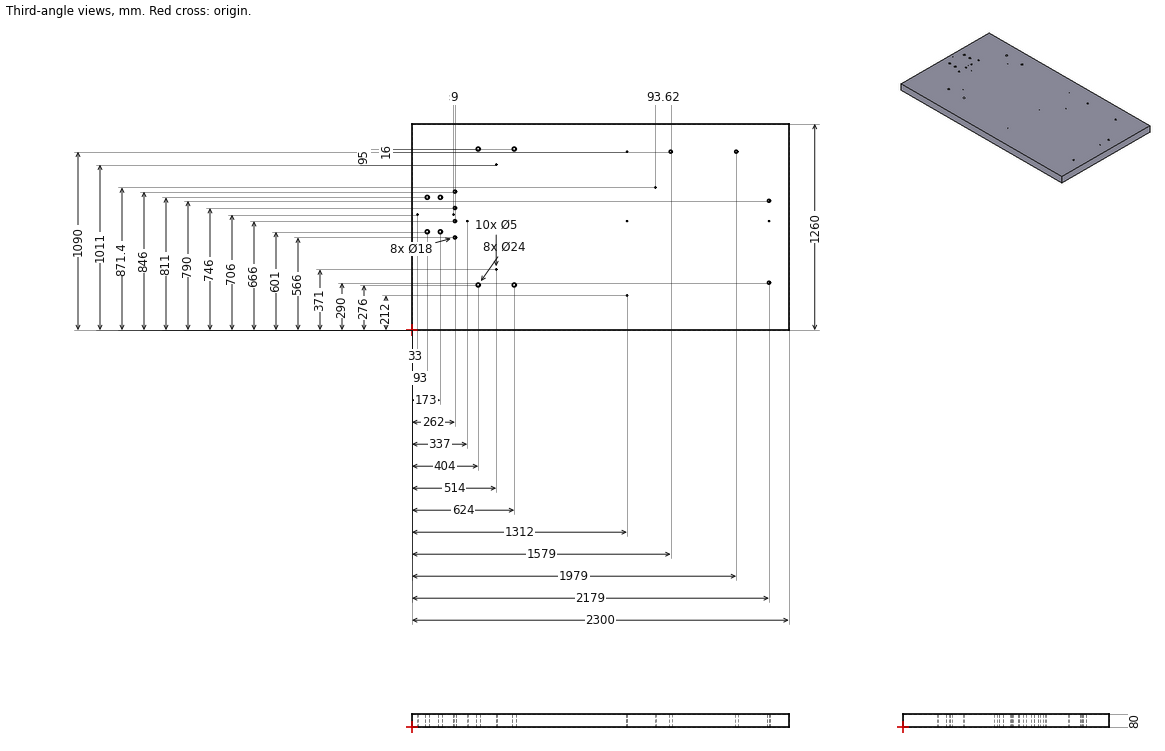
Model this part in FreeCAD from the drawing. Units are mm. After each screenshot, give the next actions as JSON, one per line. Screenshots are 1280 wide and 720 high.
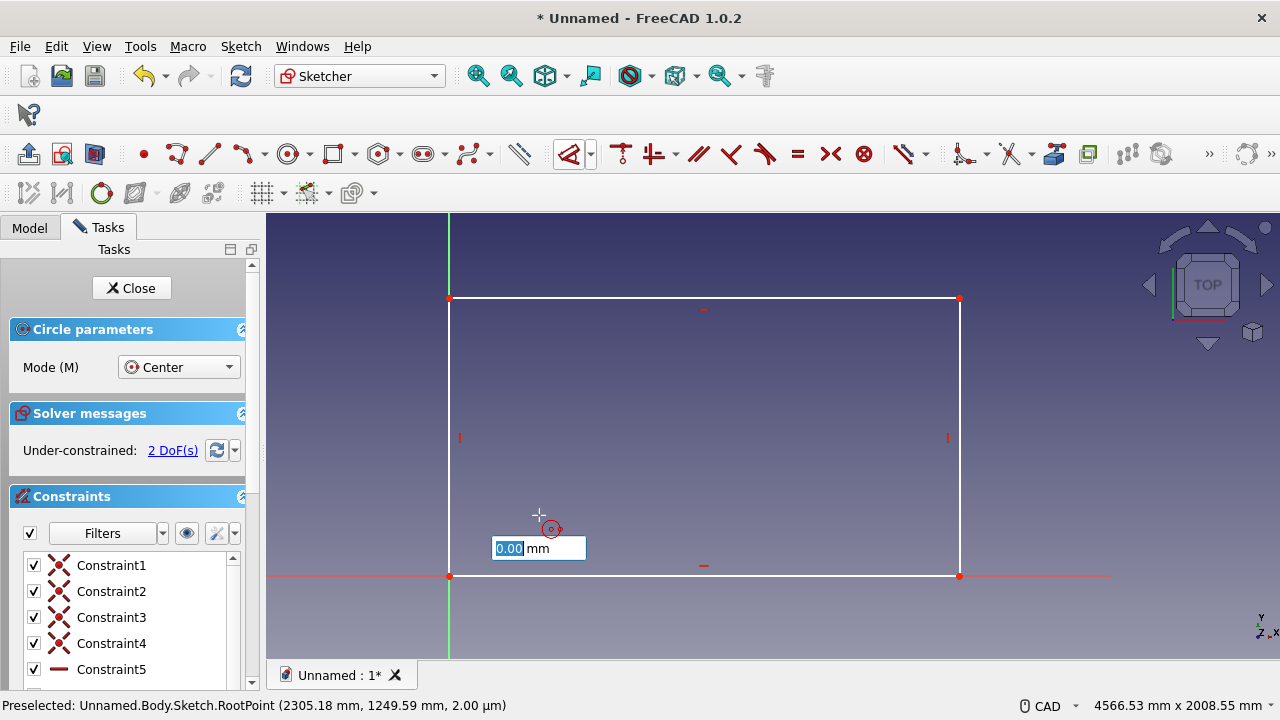
{"action": "scroll", "coordinate": [541, 513], "scroll_direction": "up", "scroll_amount": 9}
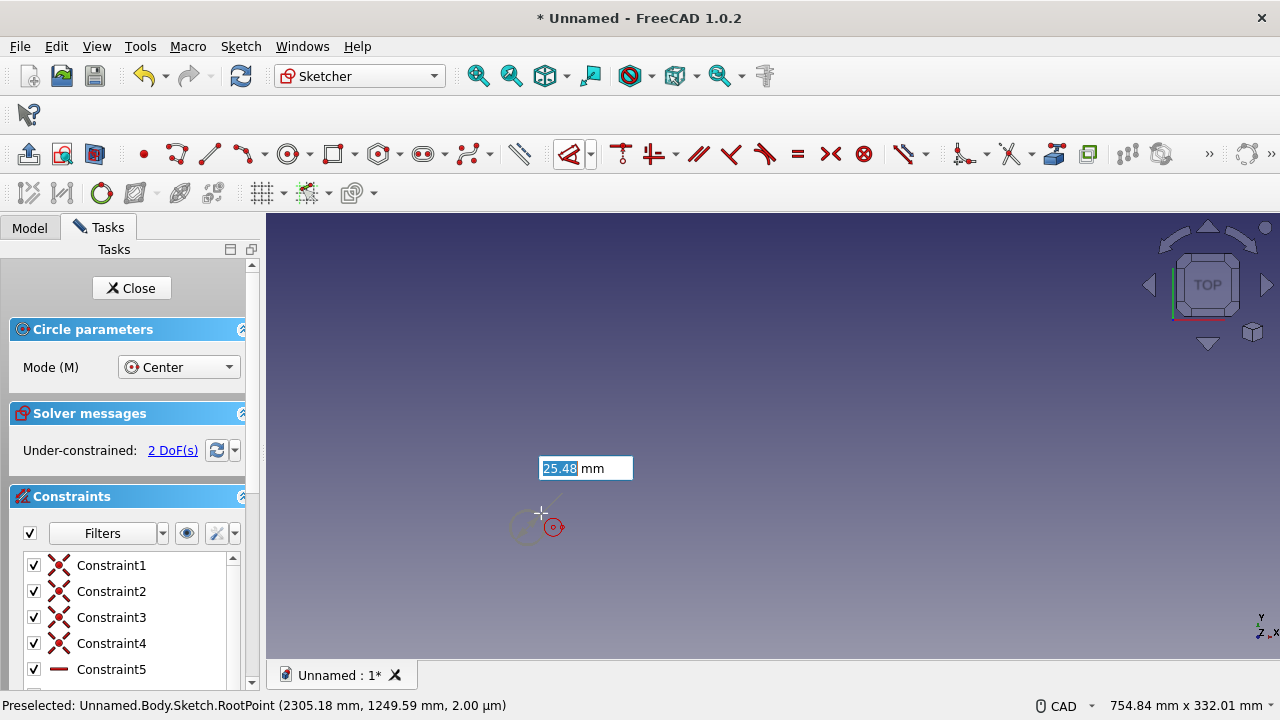
{"action": "left_click", "coordinate": [538, 511]}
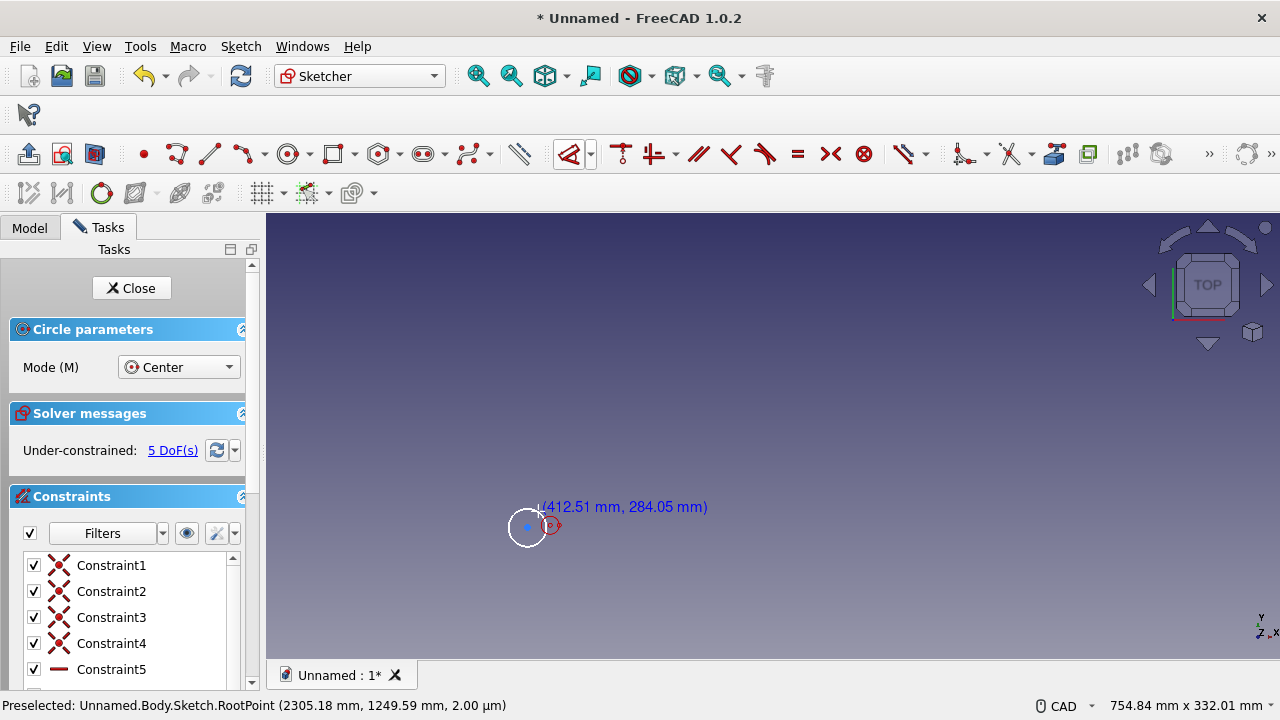
{"action": "scroll", "coordinate": [674, 395], "scroll_direction": "up", "scroll_amount": 10}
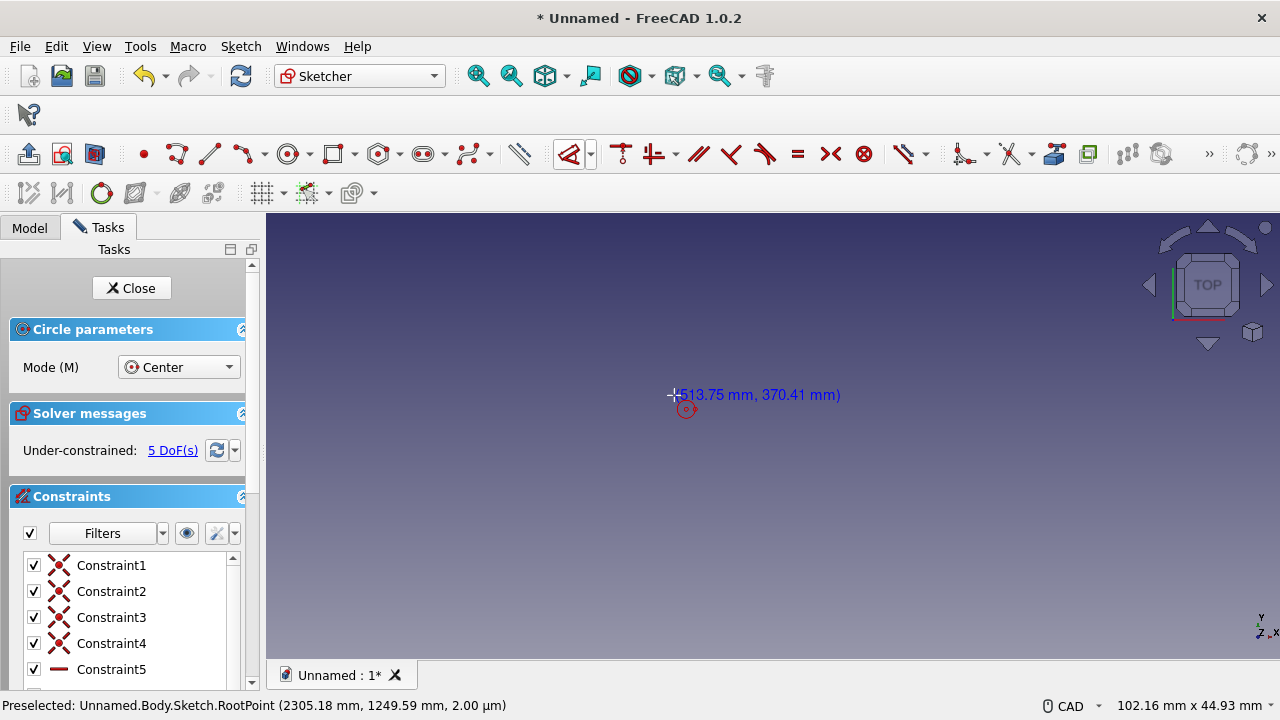
{"action": "scroll", "coordinate": [704, 436], "scroll_direction": "down", "scroll_amount": 15}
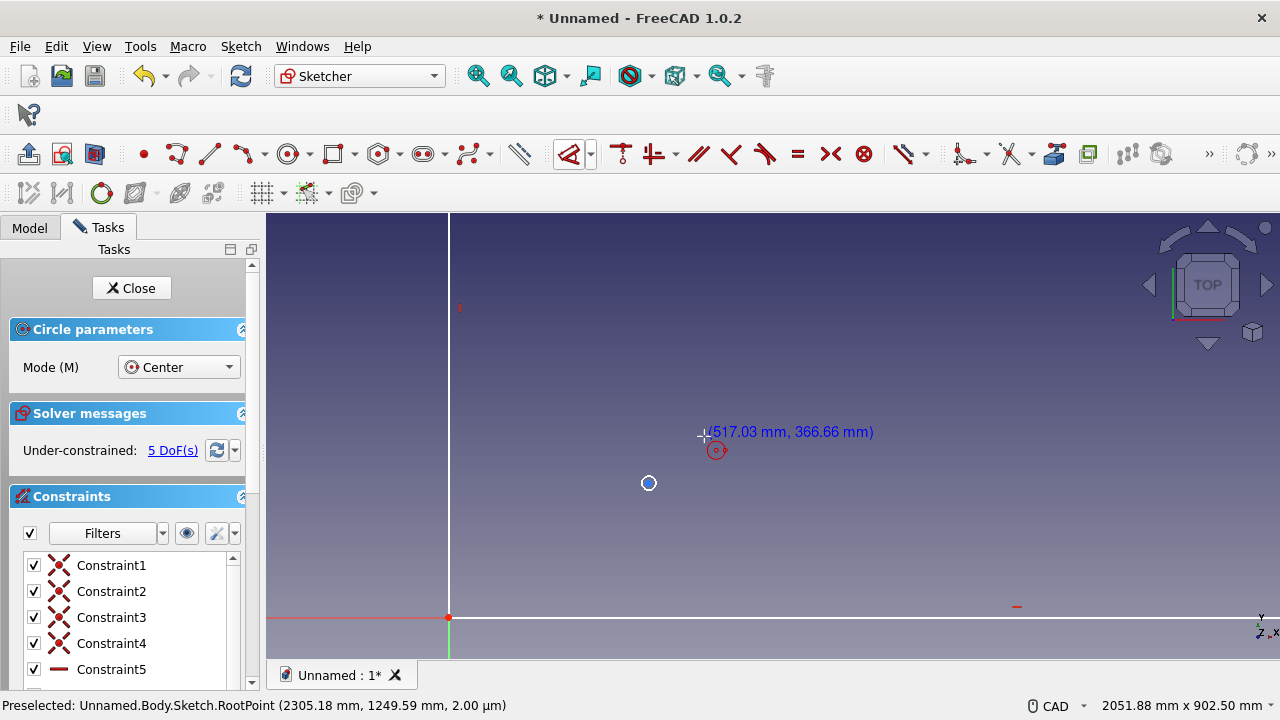
{"action": "scroll", "coordinate": [449, 542], "scroll_direction": "down", "scroll_amount": 4}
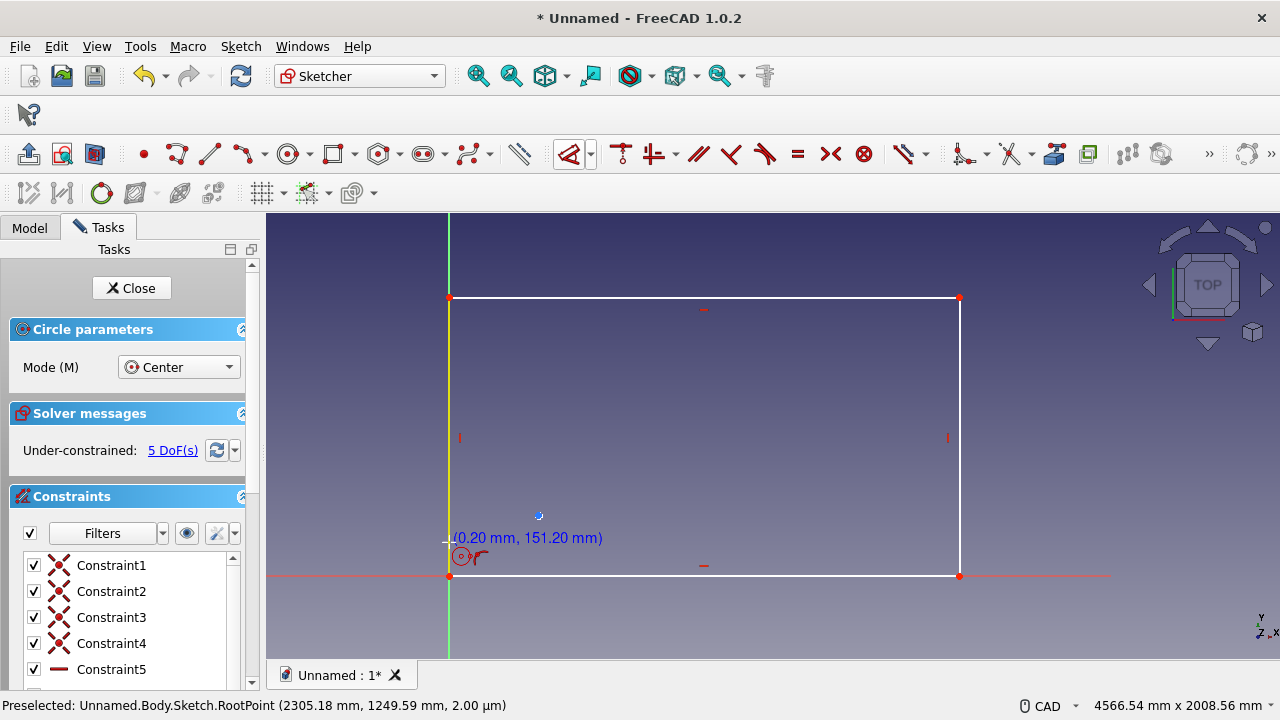
{"action": "left_click", "coordinate": [563, 494]}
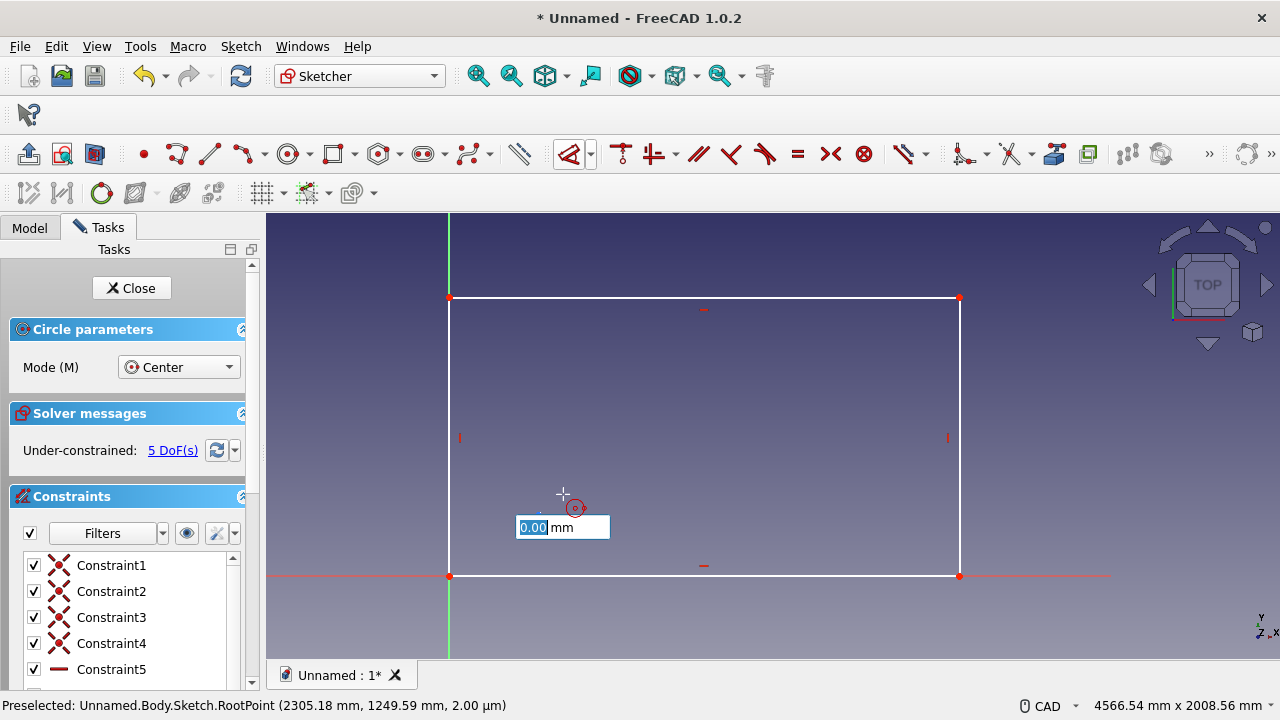
{"action": "scroll", "coordinate": [564, 494], "scroll_direction": "up", "scroll_amount": 17}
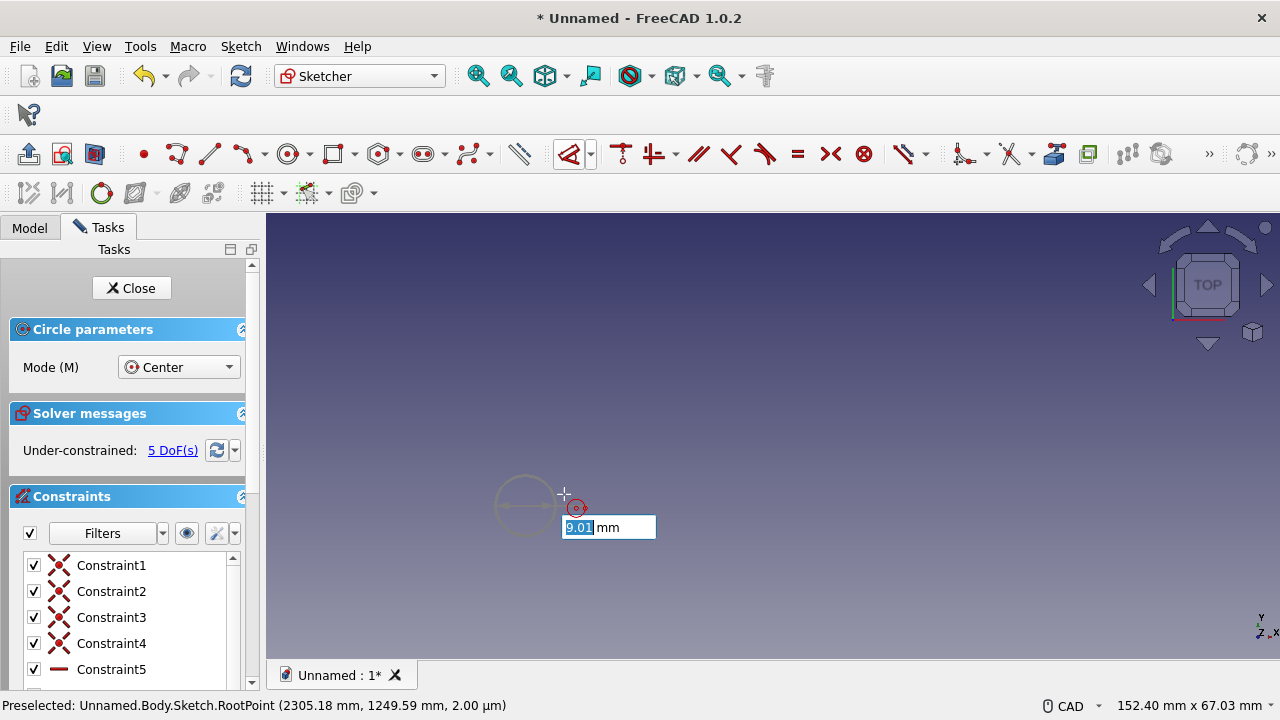
{"action": "left_click", "coordinate": [543, 465]}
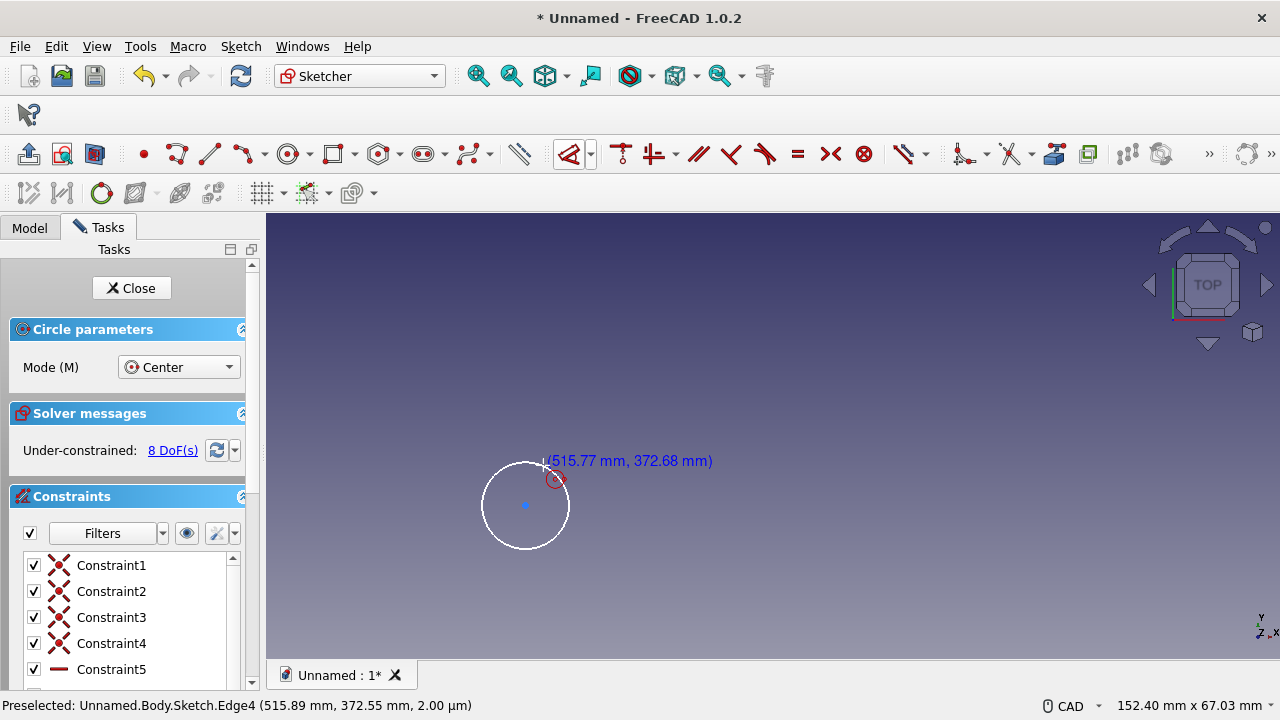
{"action": "scroll", "coordinate": [564, 494], "scroll_direction": "down", "scroll_amount": 17}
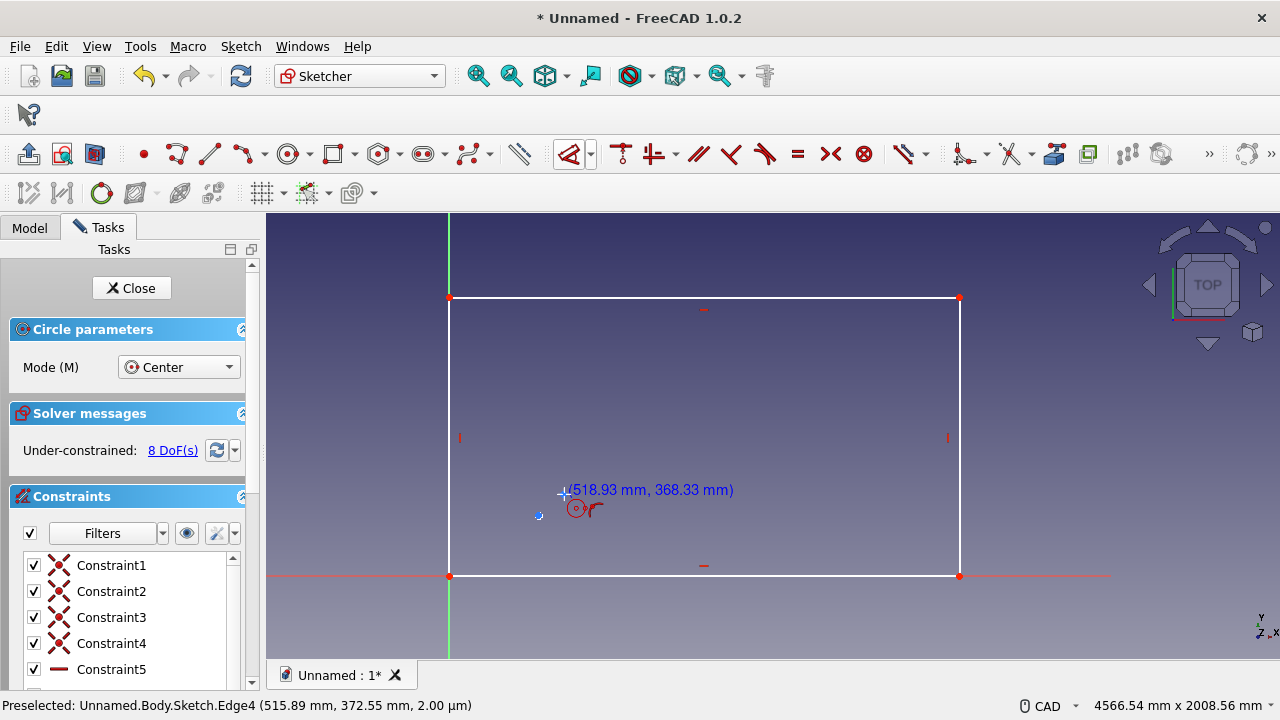
{"action": "scroll", "coordinate": [588, 515], "scroll_direction": "up", "scroll_amount": 11}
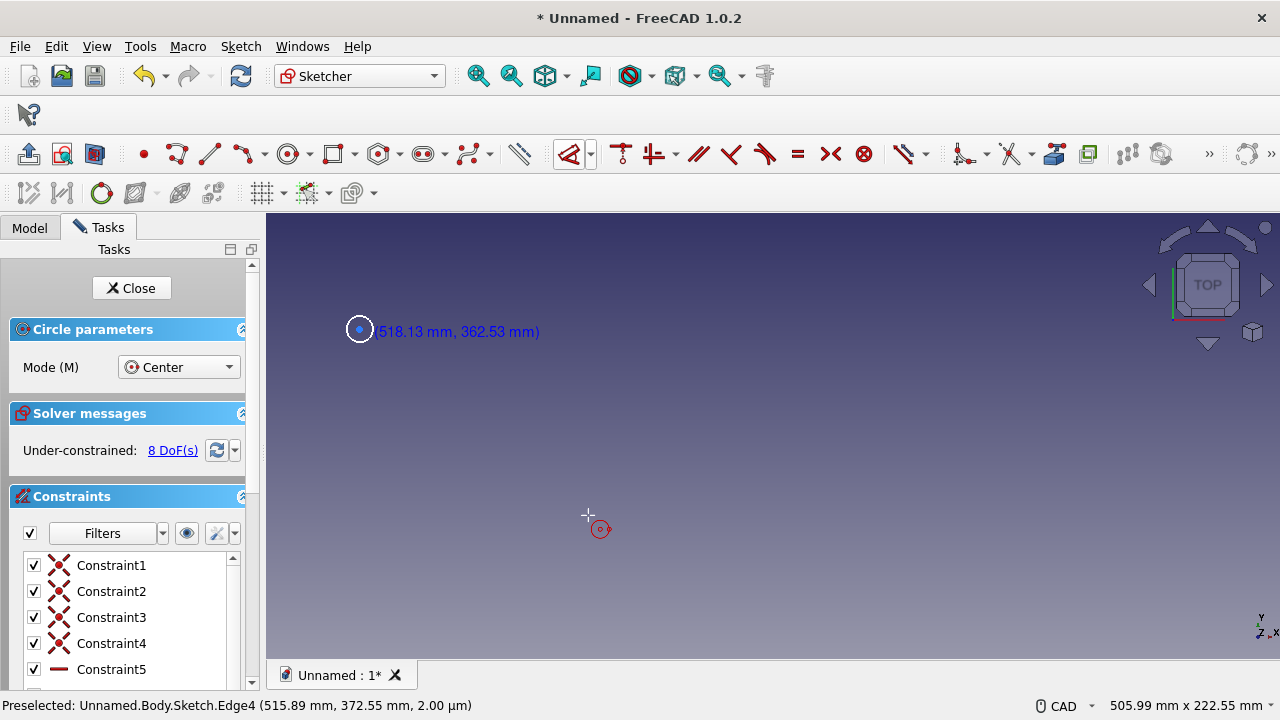
{"action": "scroll", "coordinate": [588, 515], "scroll_direction": "down", "scroll_amount": 11}